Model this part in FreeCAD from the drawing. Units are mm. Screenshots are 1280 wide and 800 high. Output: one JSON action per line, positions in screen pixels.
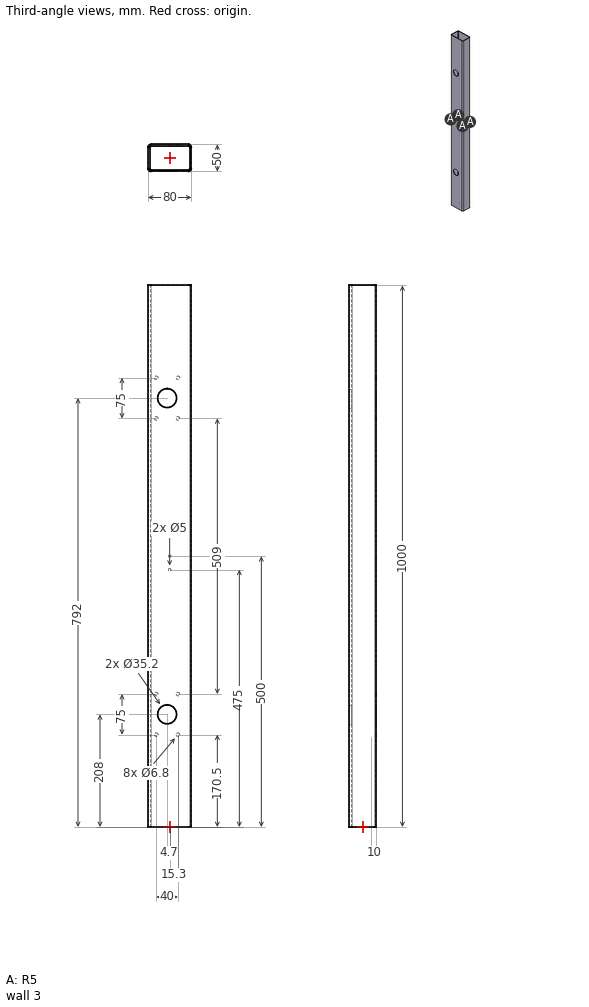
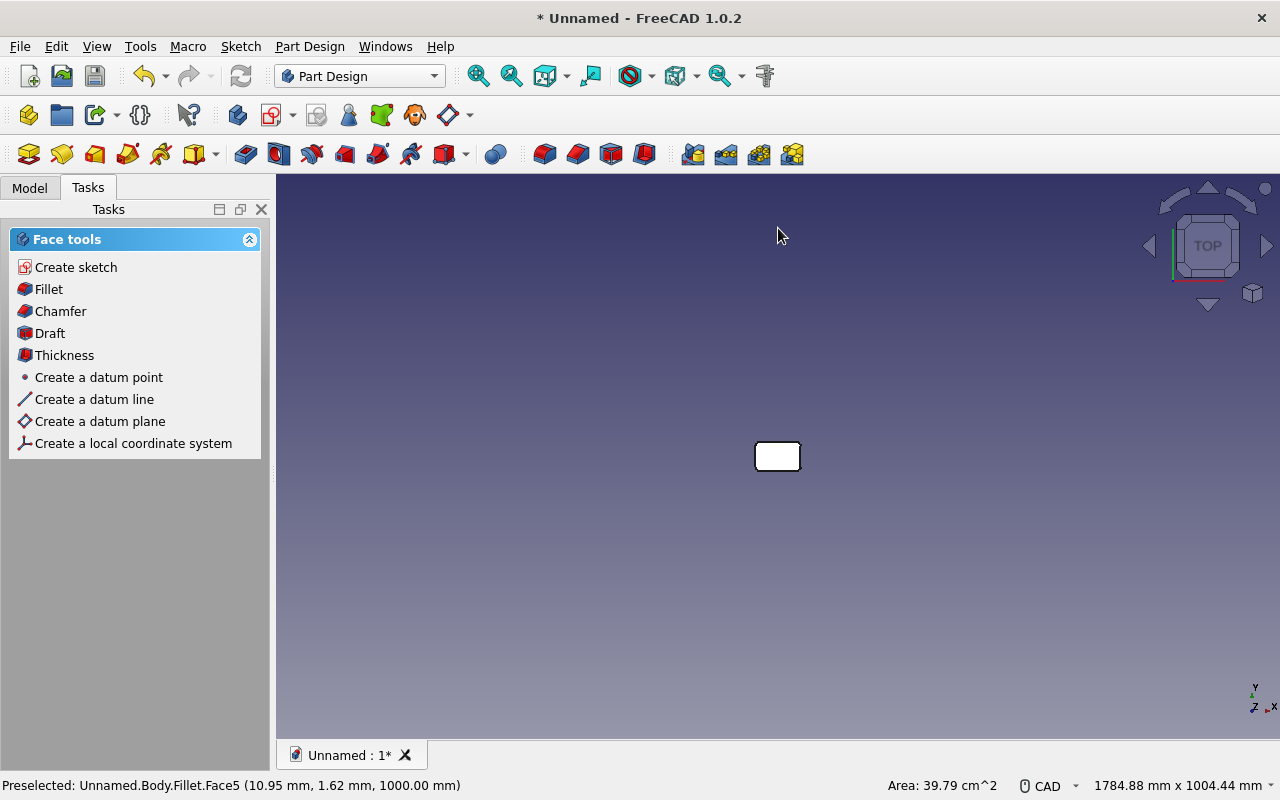
{"action": "left_click", "coordinate": [479, 76]}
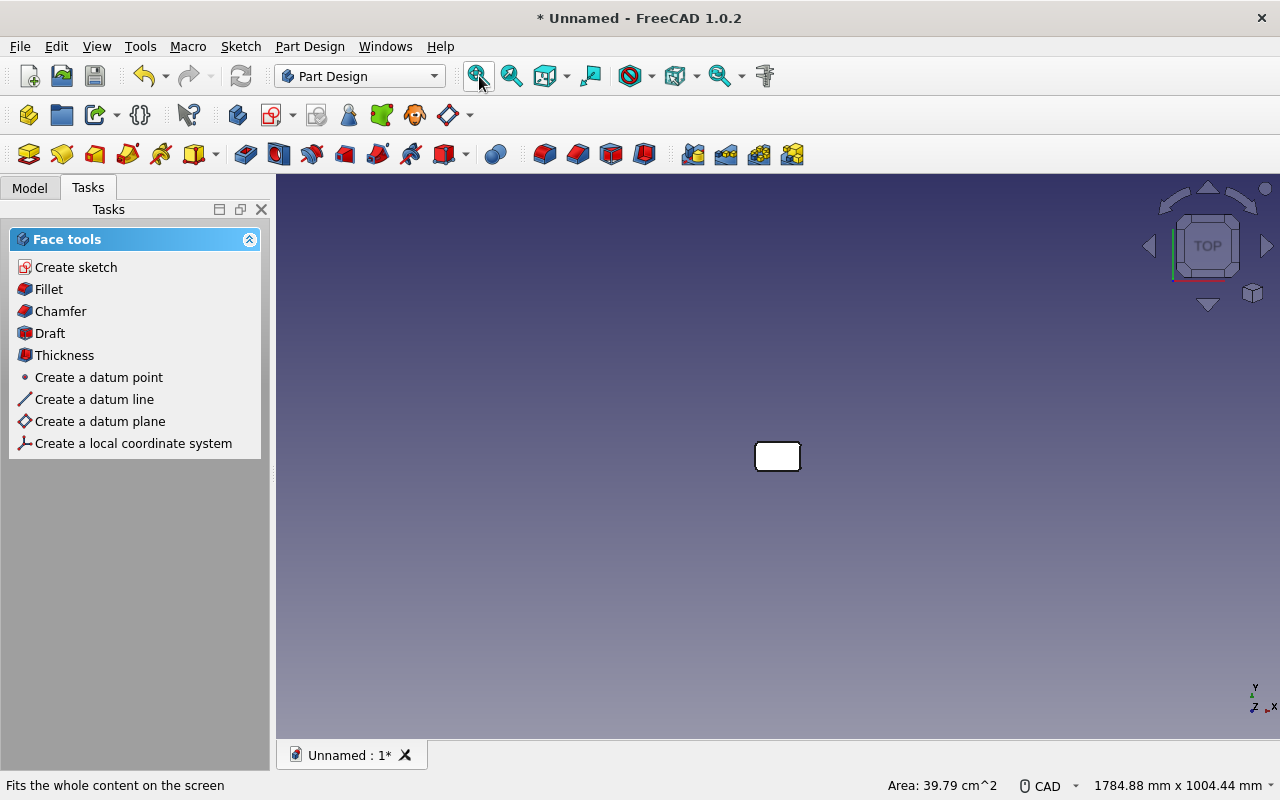
{"action": "key", "text": "1"}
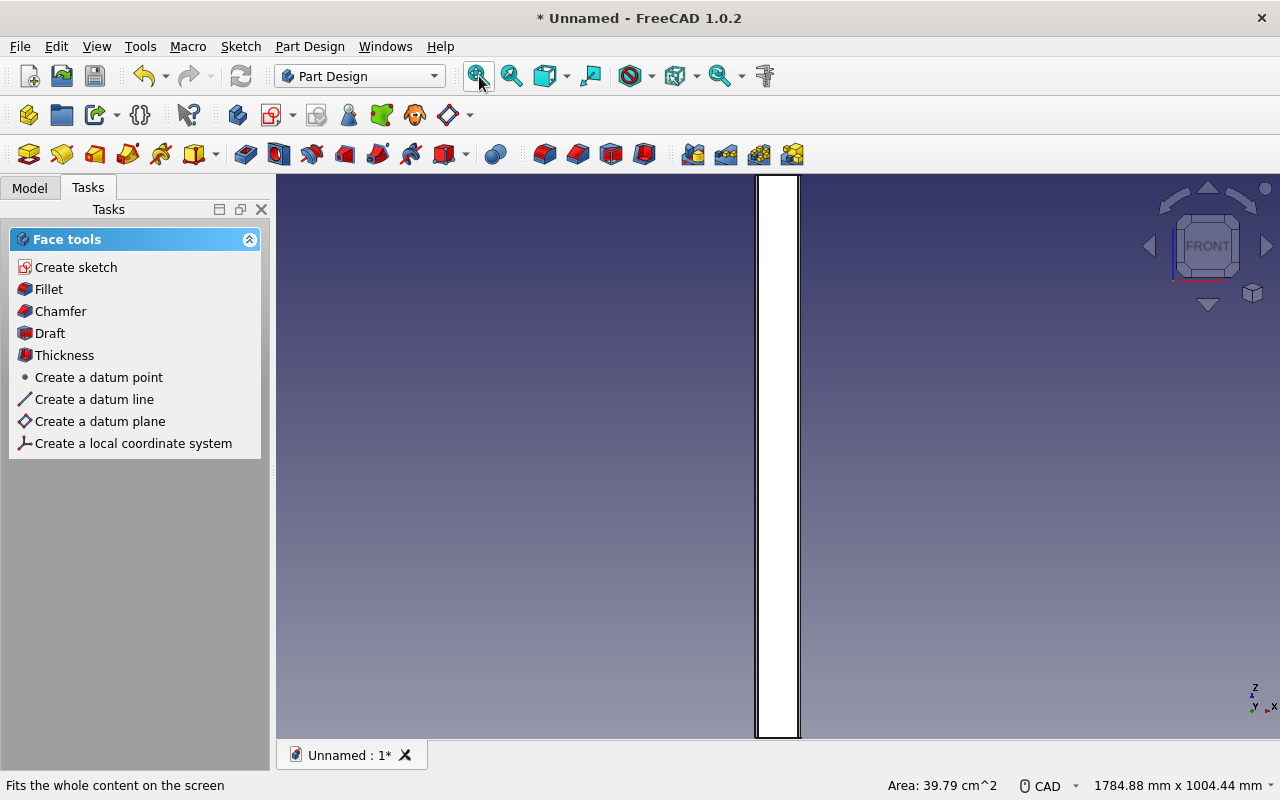
{"action": "key", "text": "3"}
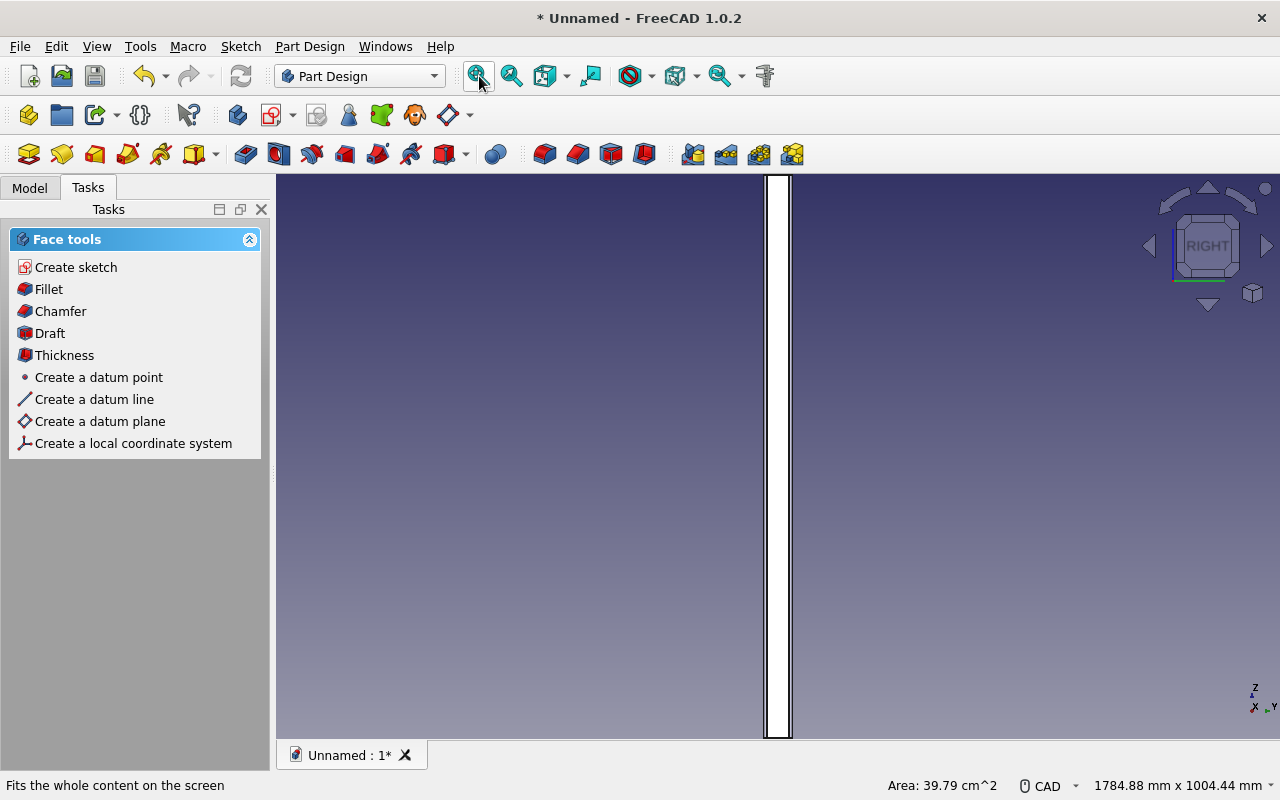
{"action": "key", "text": "5"}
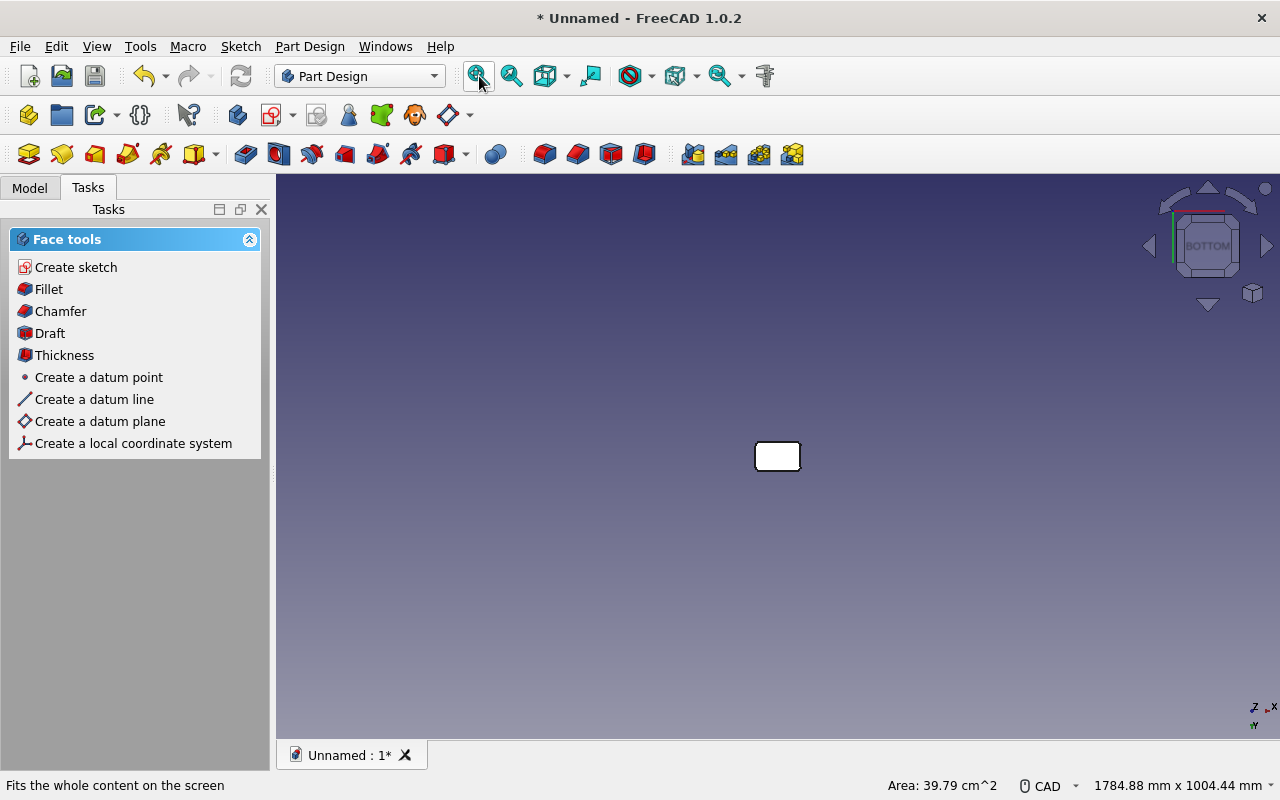
{"action": "left_click", "coordinate": [479, 76]}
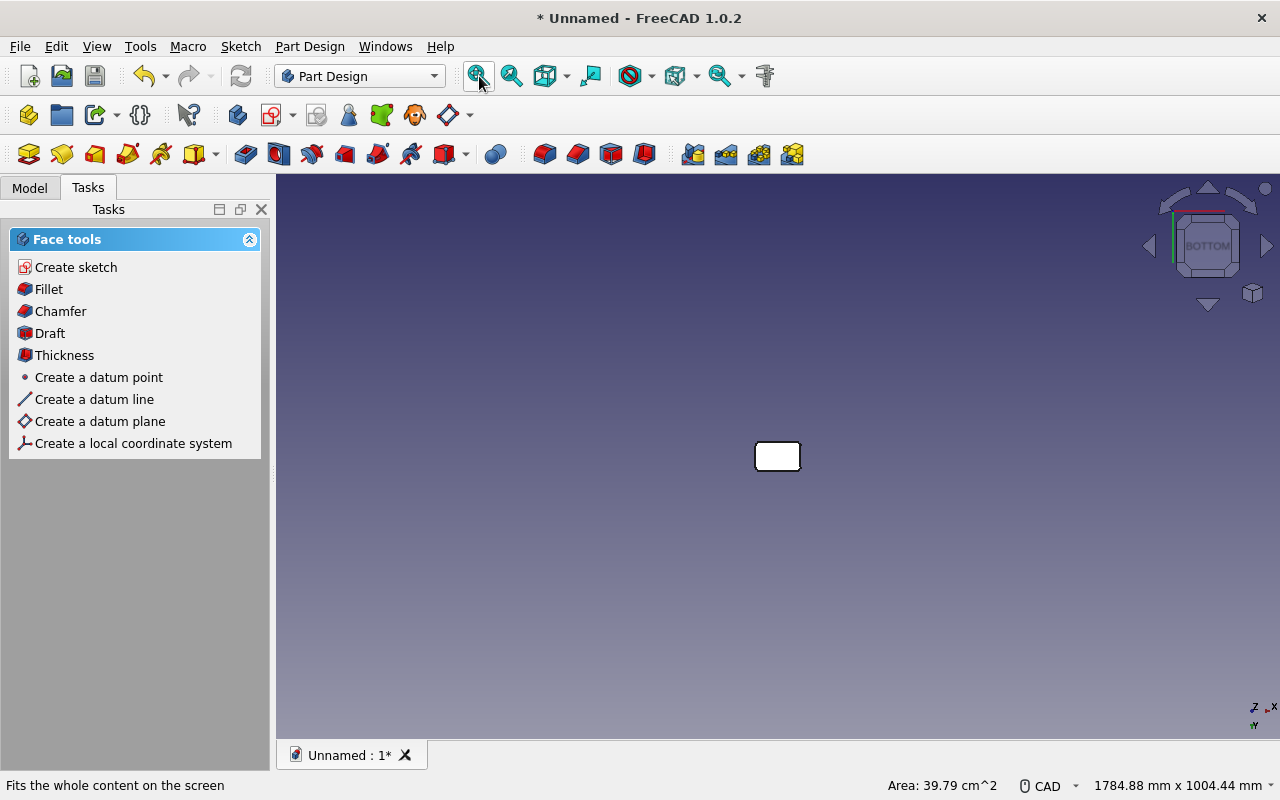
{"action": "left_click", "coordinate": [784, 455], "text": "ctrl"}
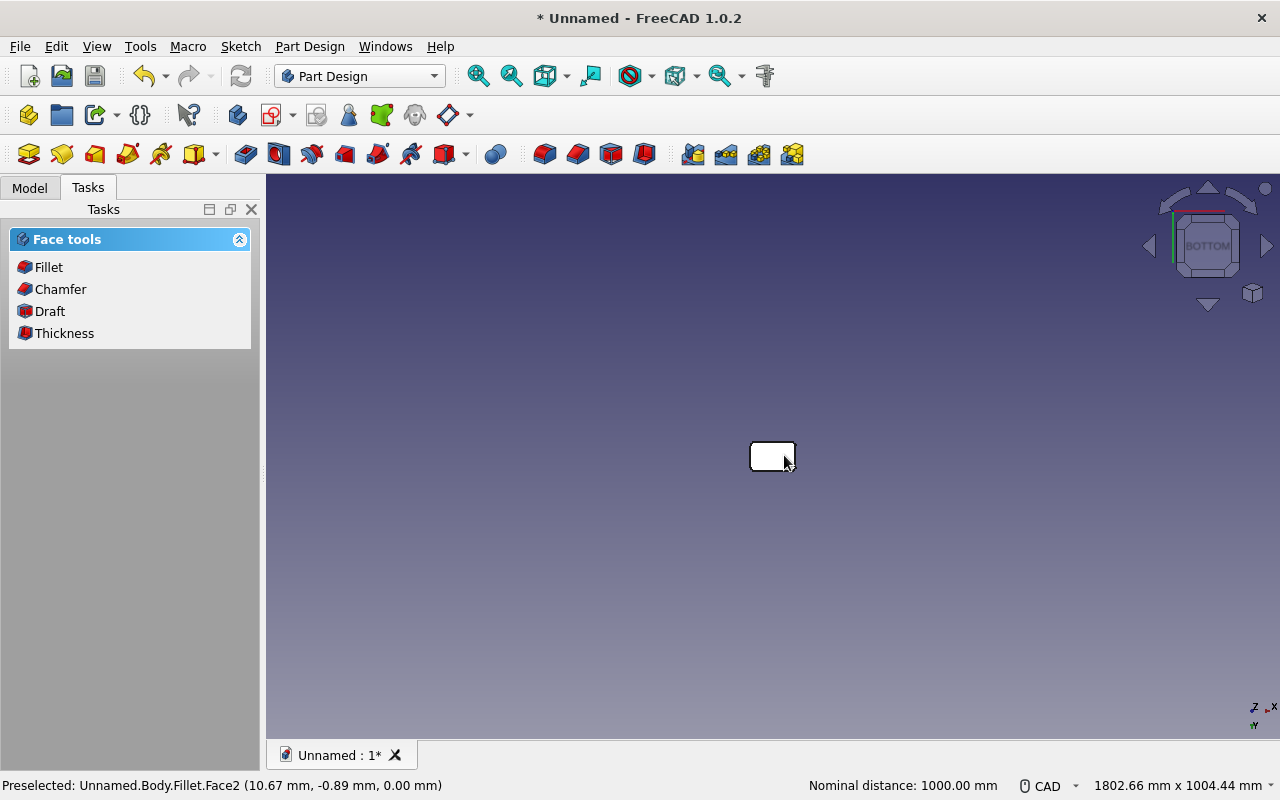
{"action": "left_click", "coordinate": [644, 154]}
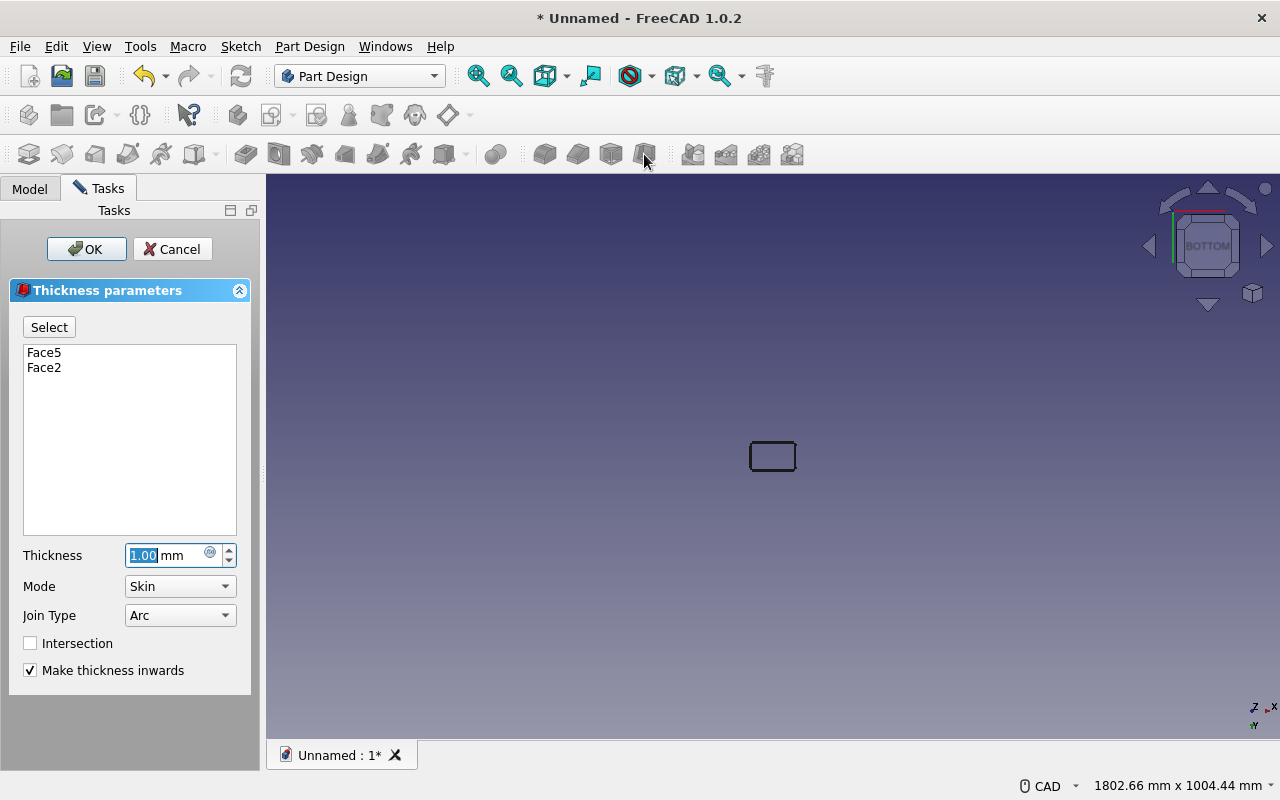
{"action": "type", "text": "3"}
{"action": "key", "text": "Tab"}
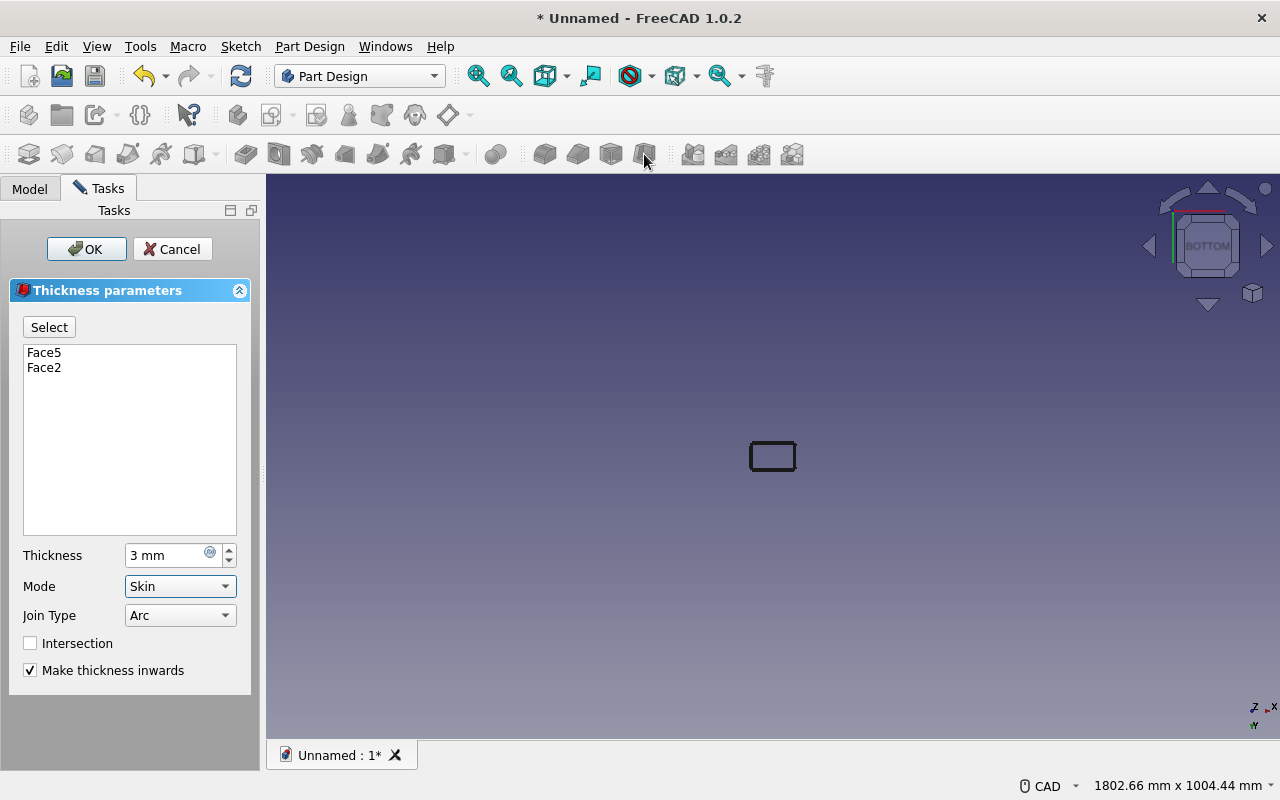
{"action": "left_click", "coordinate": [181, 616]}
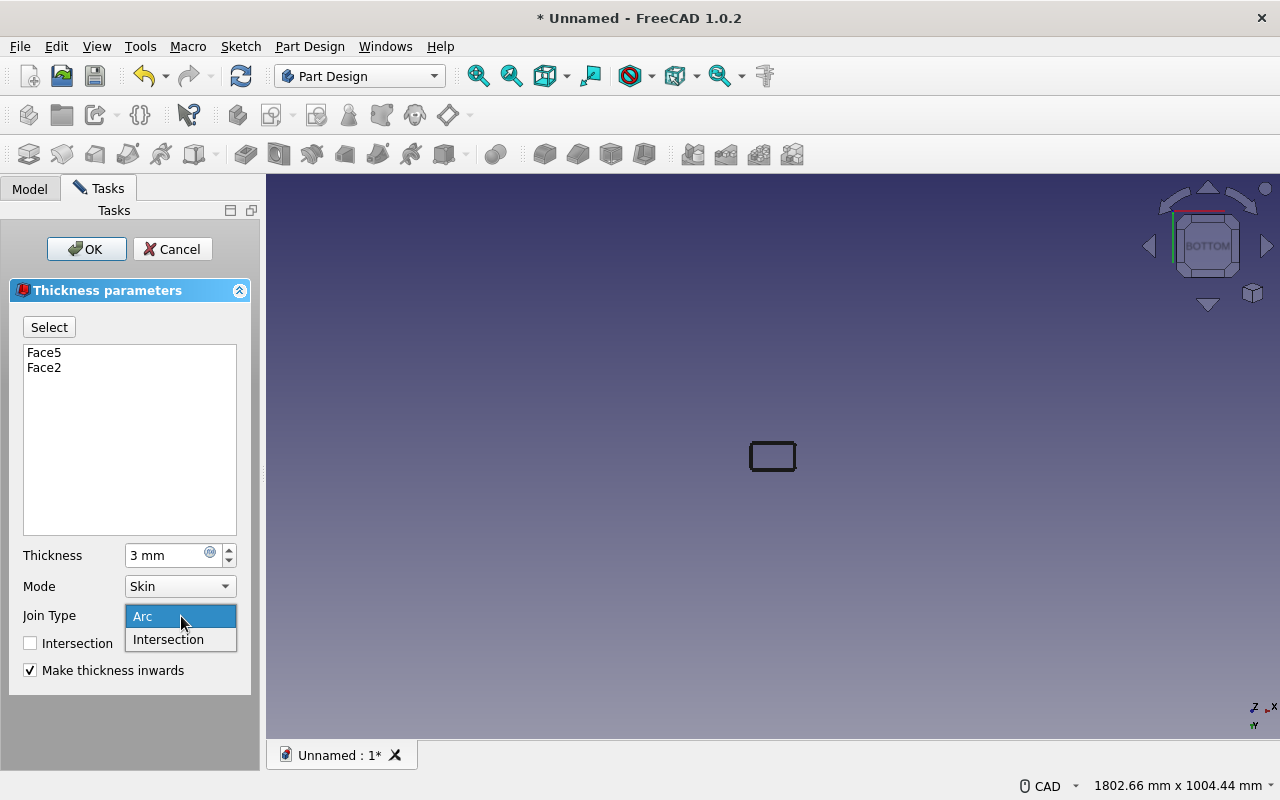
{"action": "left_click", "coordinate": [179, 640]}